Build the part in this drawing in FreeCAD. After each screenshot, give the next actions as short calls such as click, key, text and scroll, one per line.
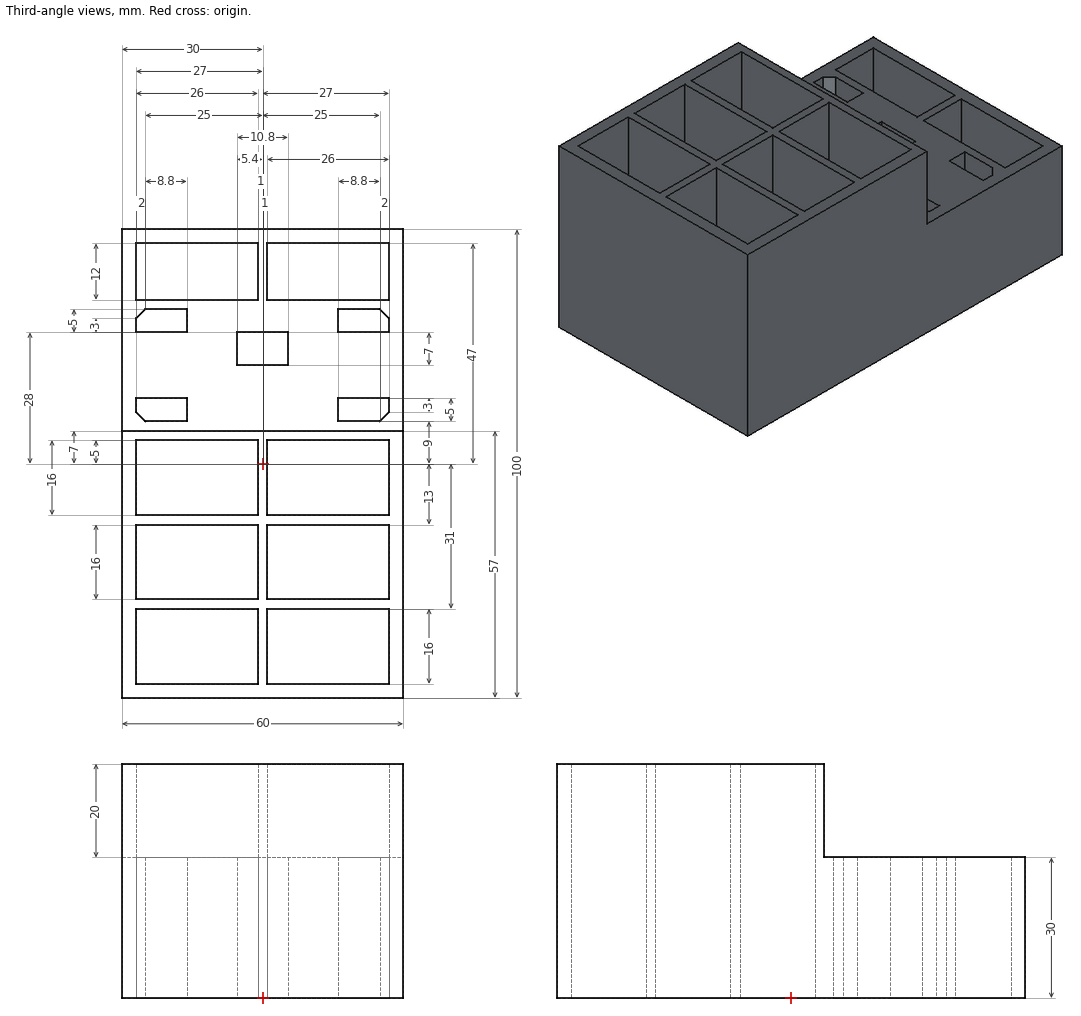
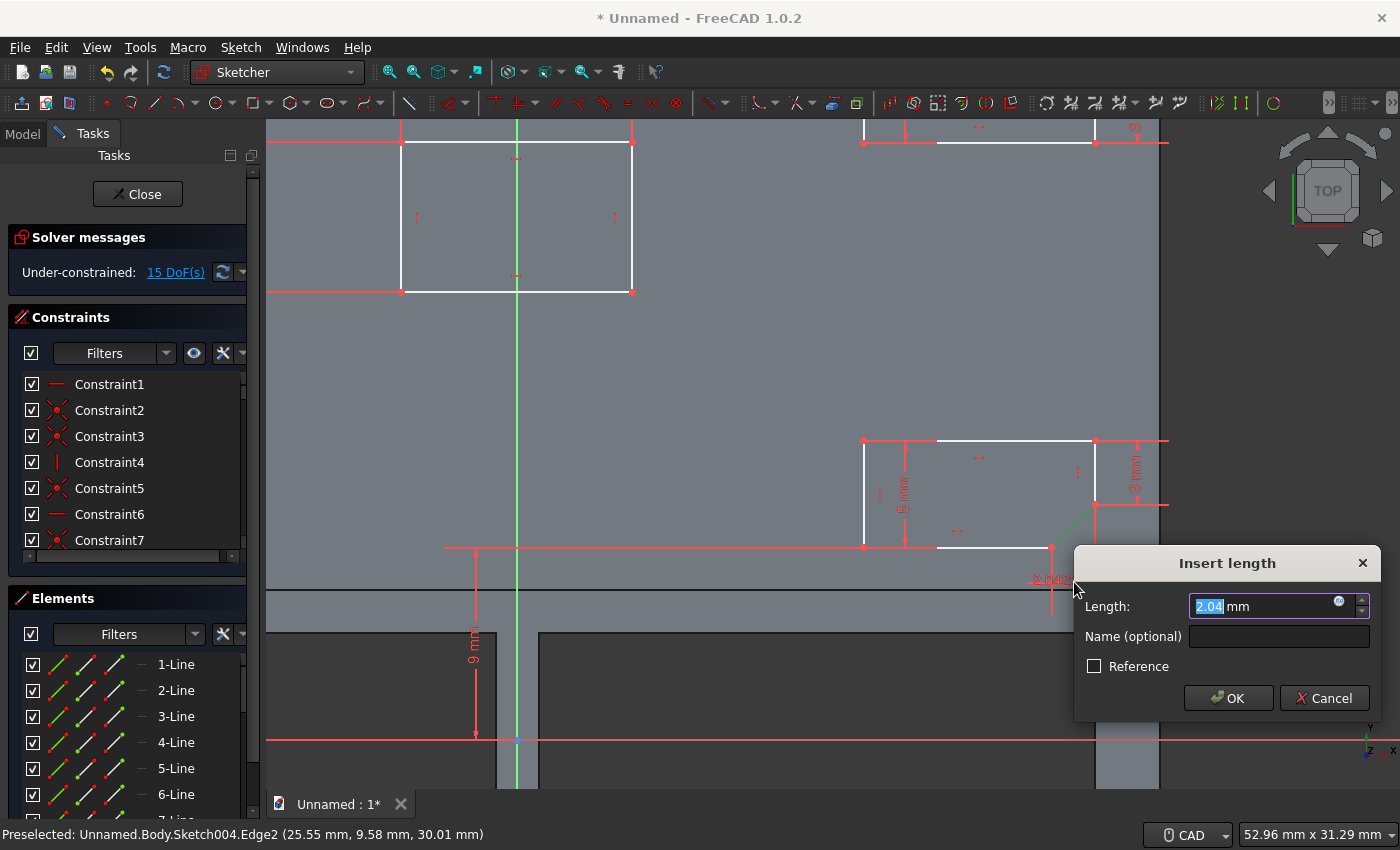
text(2)
key(Return)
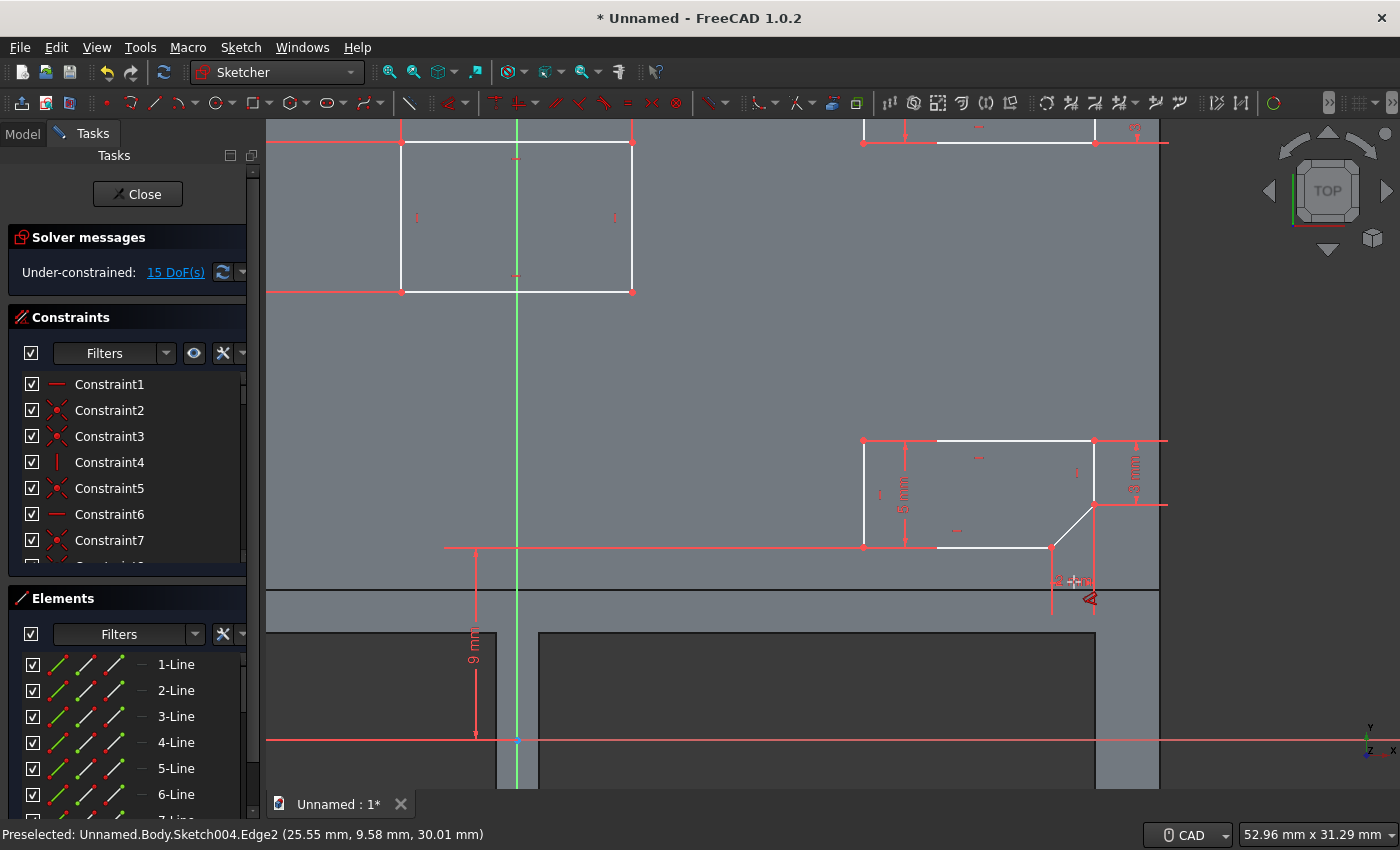
scroll(1065, 535, down, 3)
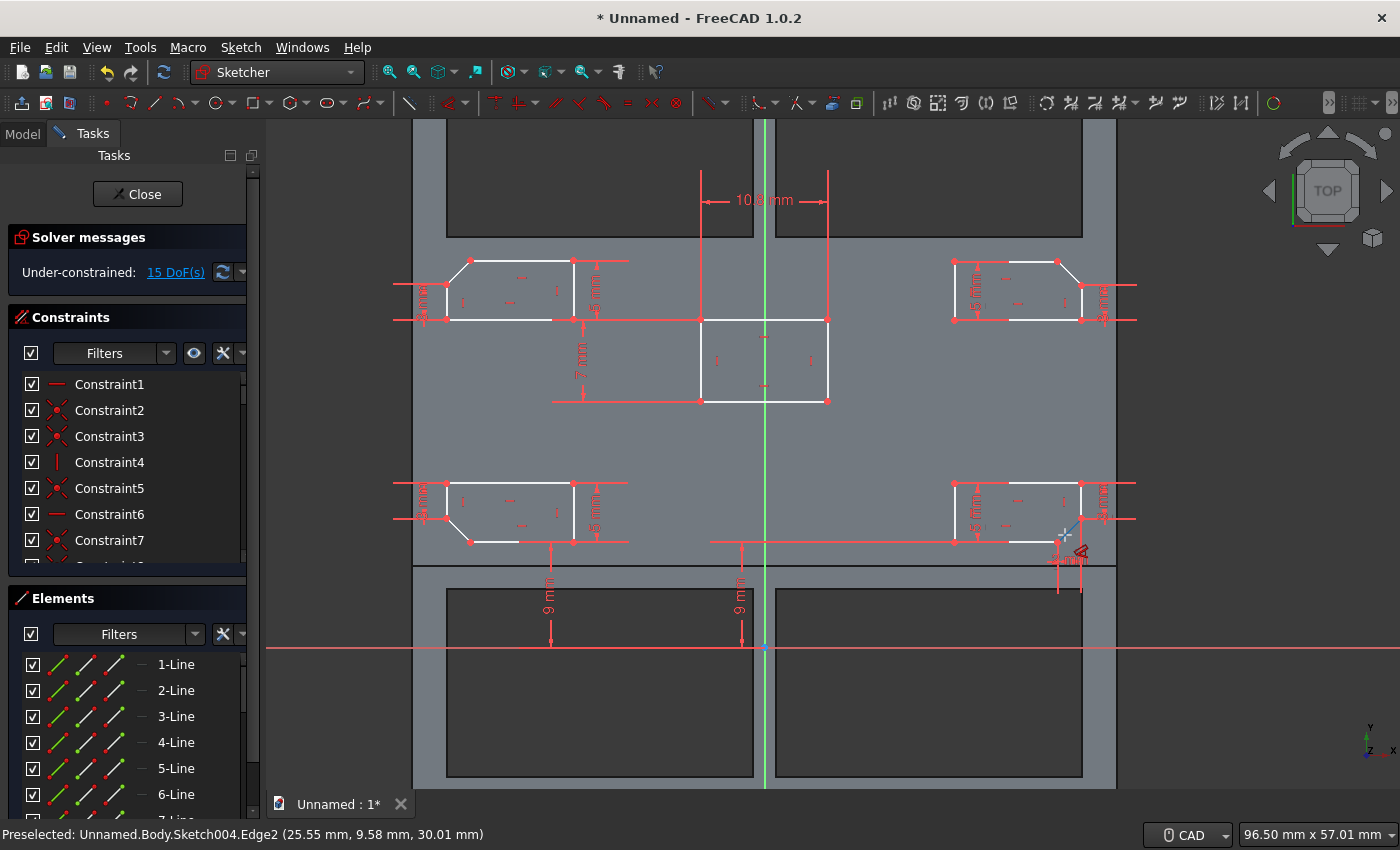
scroll(464, 268, up, 3)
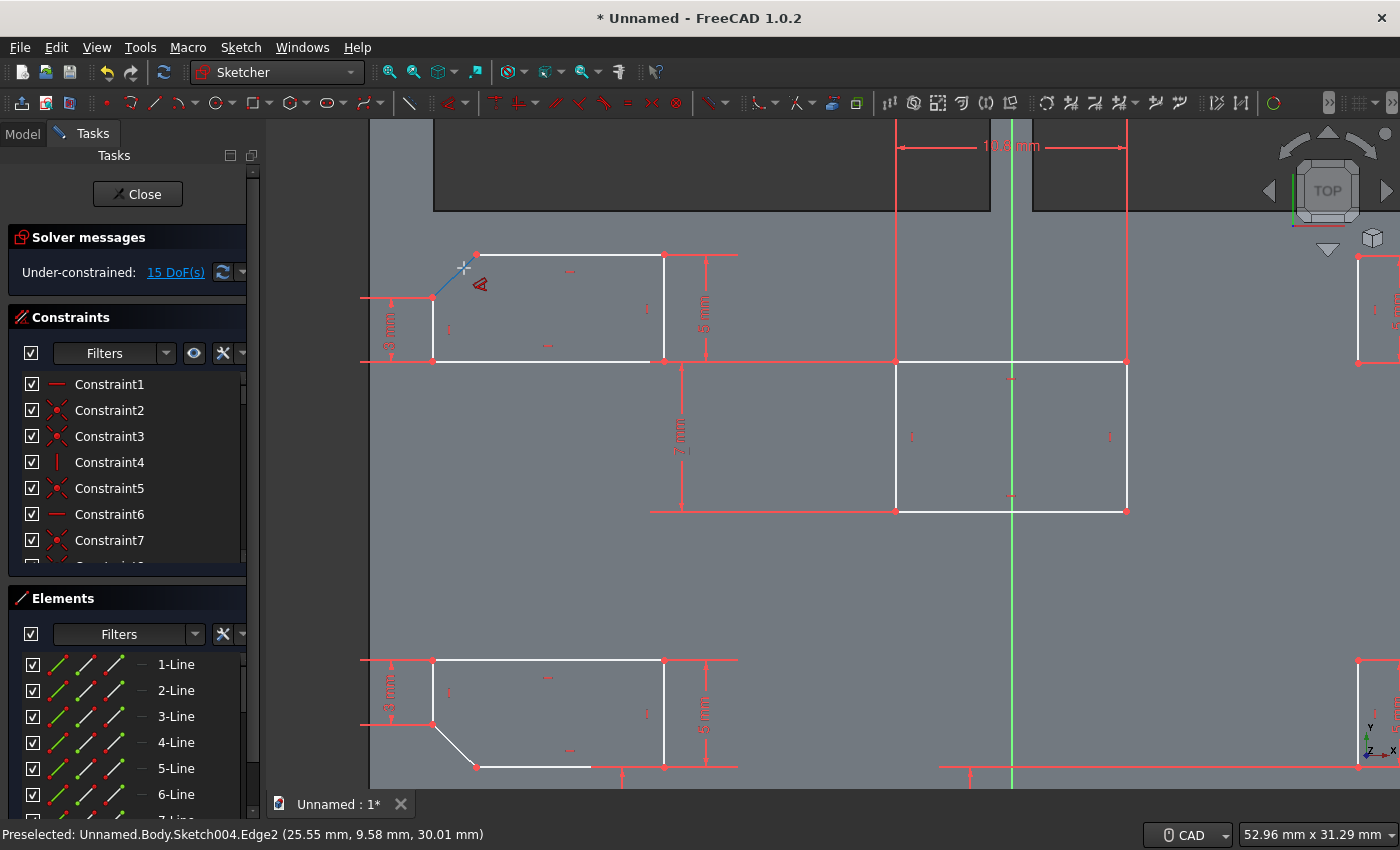
click(463, 268)
click(455, 221)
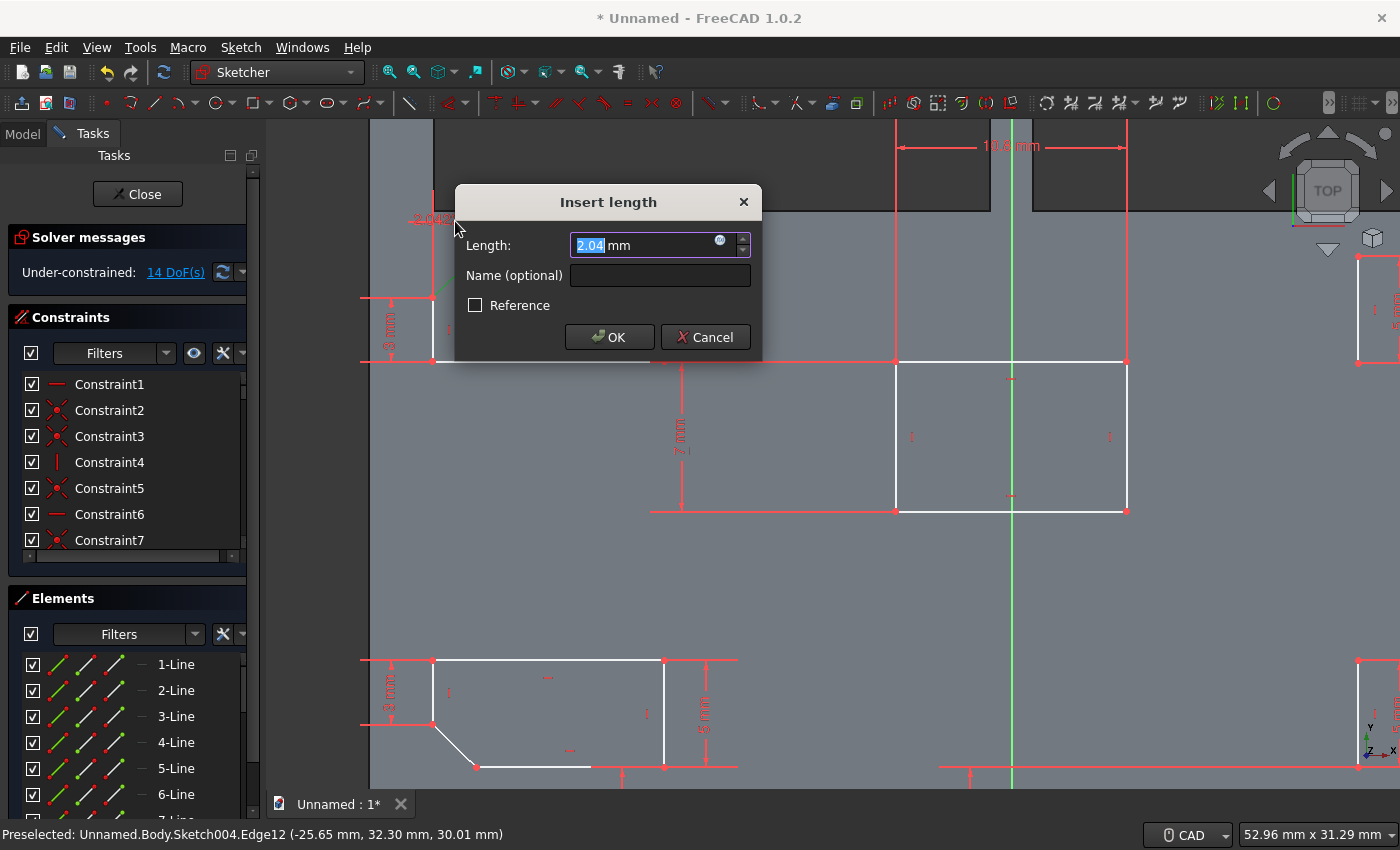
text(2)
key(Return)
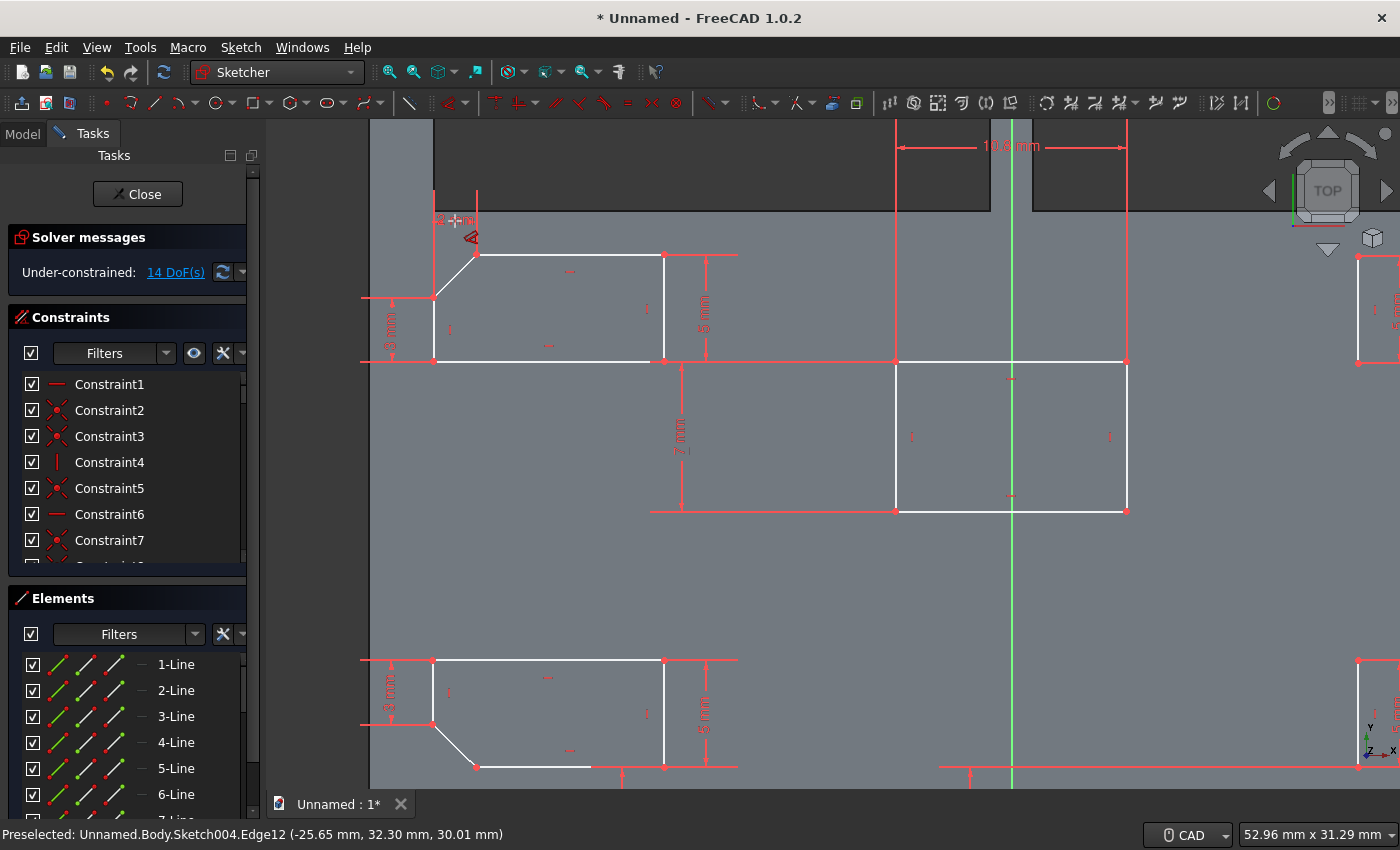
scroll(464, 268, down, 3)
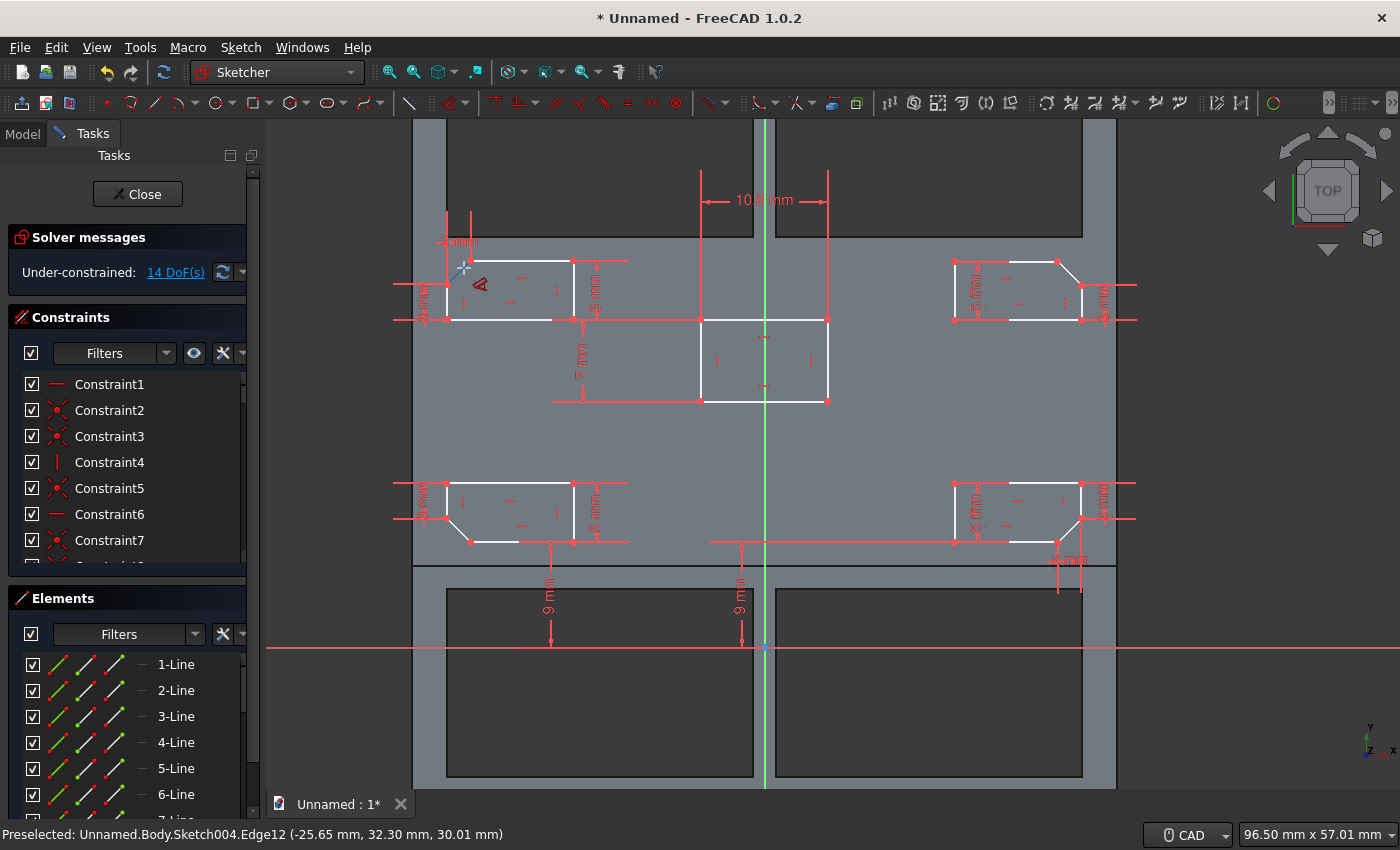
scroll(1075, 278, up, 3)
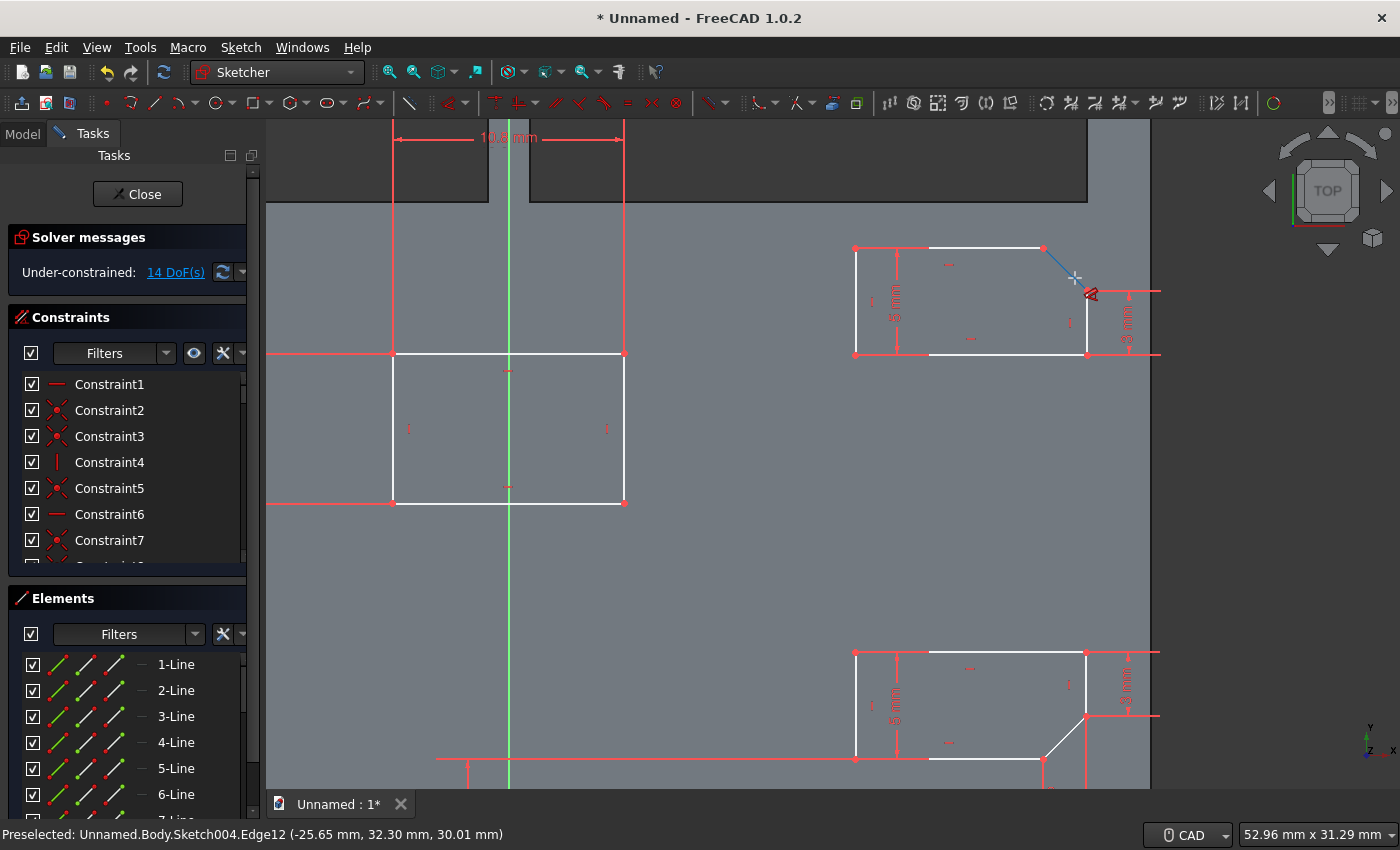
click(1074, 278)
click(1065, 214)